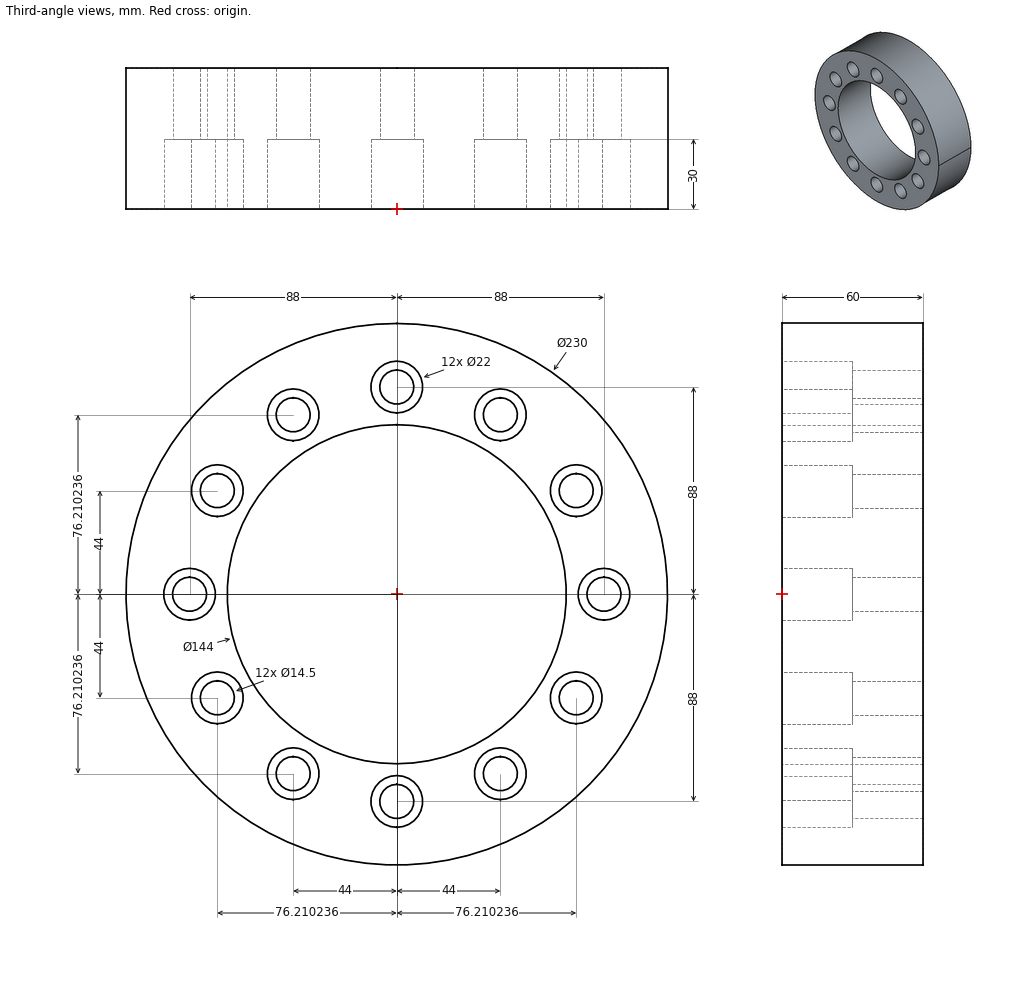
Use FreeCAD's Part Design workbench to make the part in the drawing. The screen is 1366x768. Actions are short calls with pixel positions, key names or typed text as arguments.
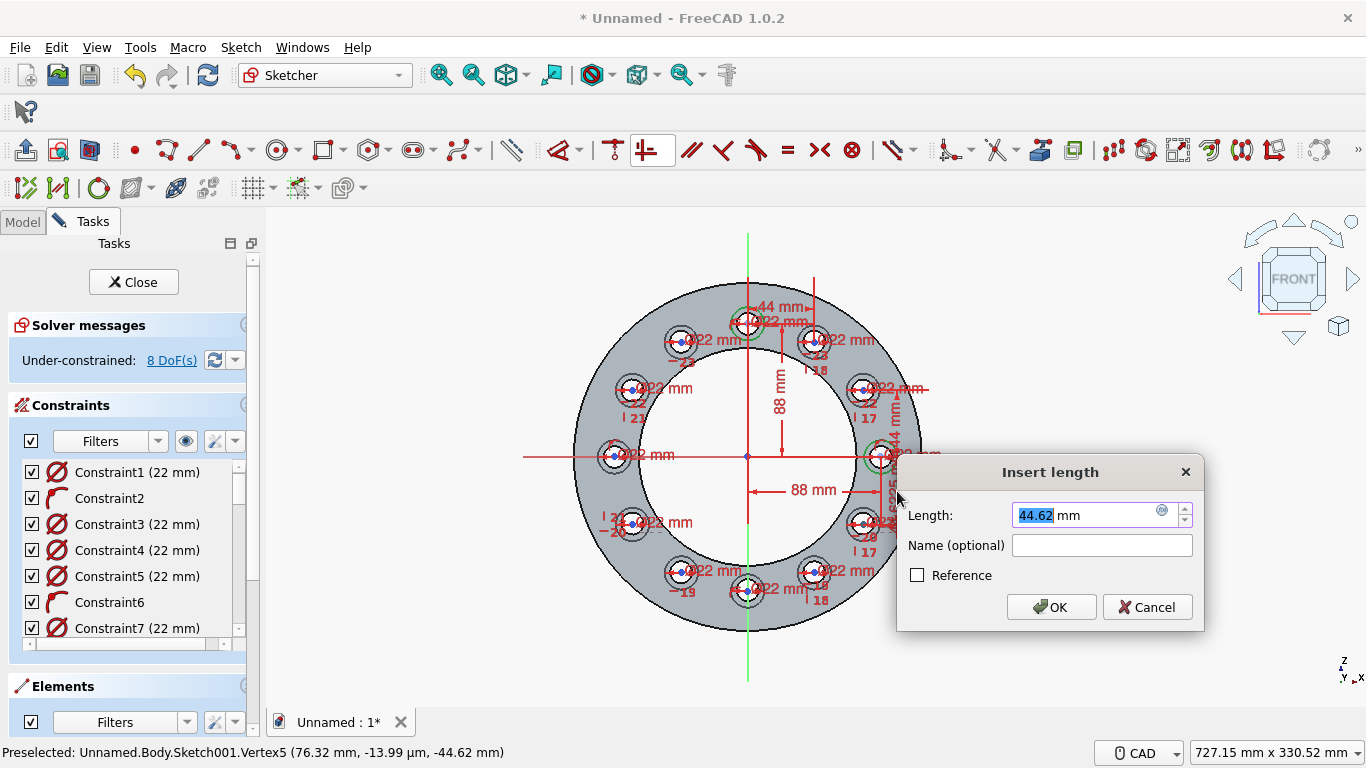
text(44)
key(Return)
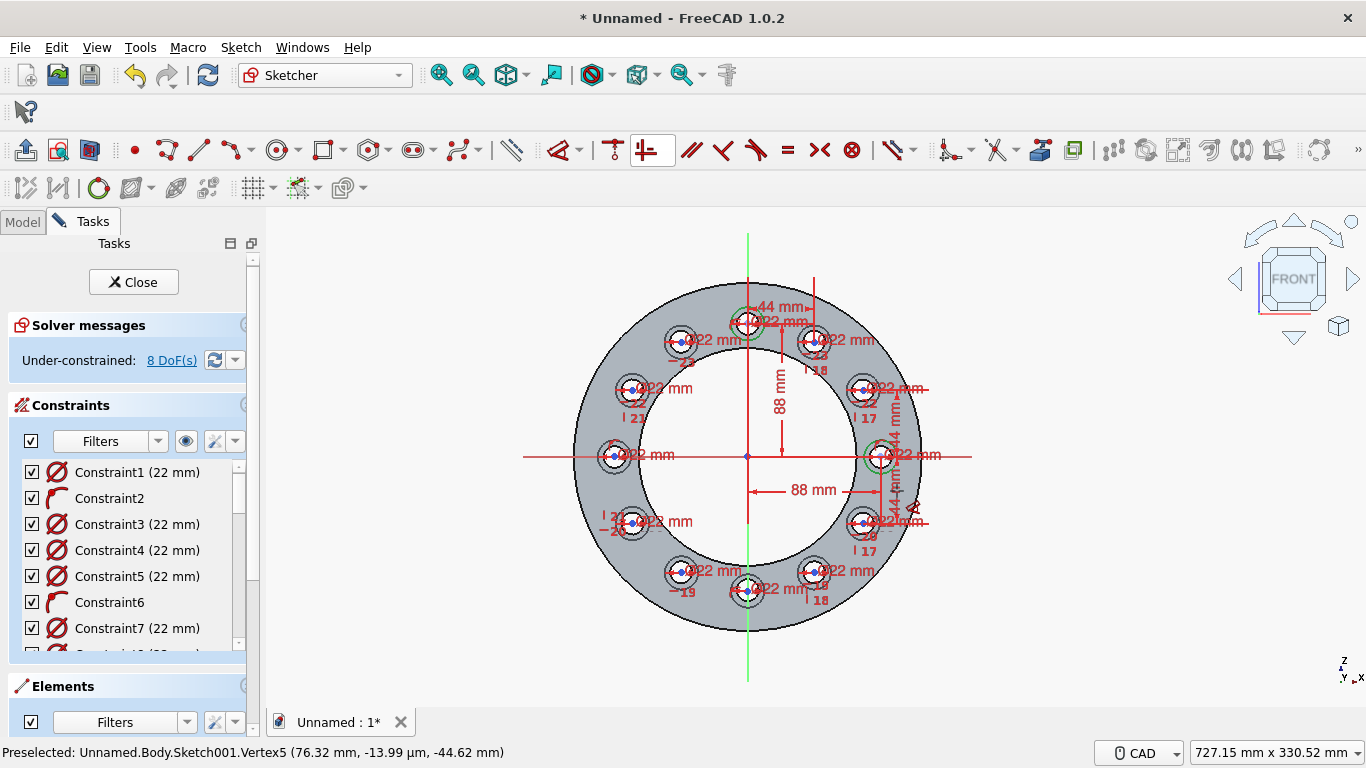
click(748, 591)
click(782, 524)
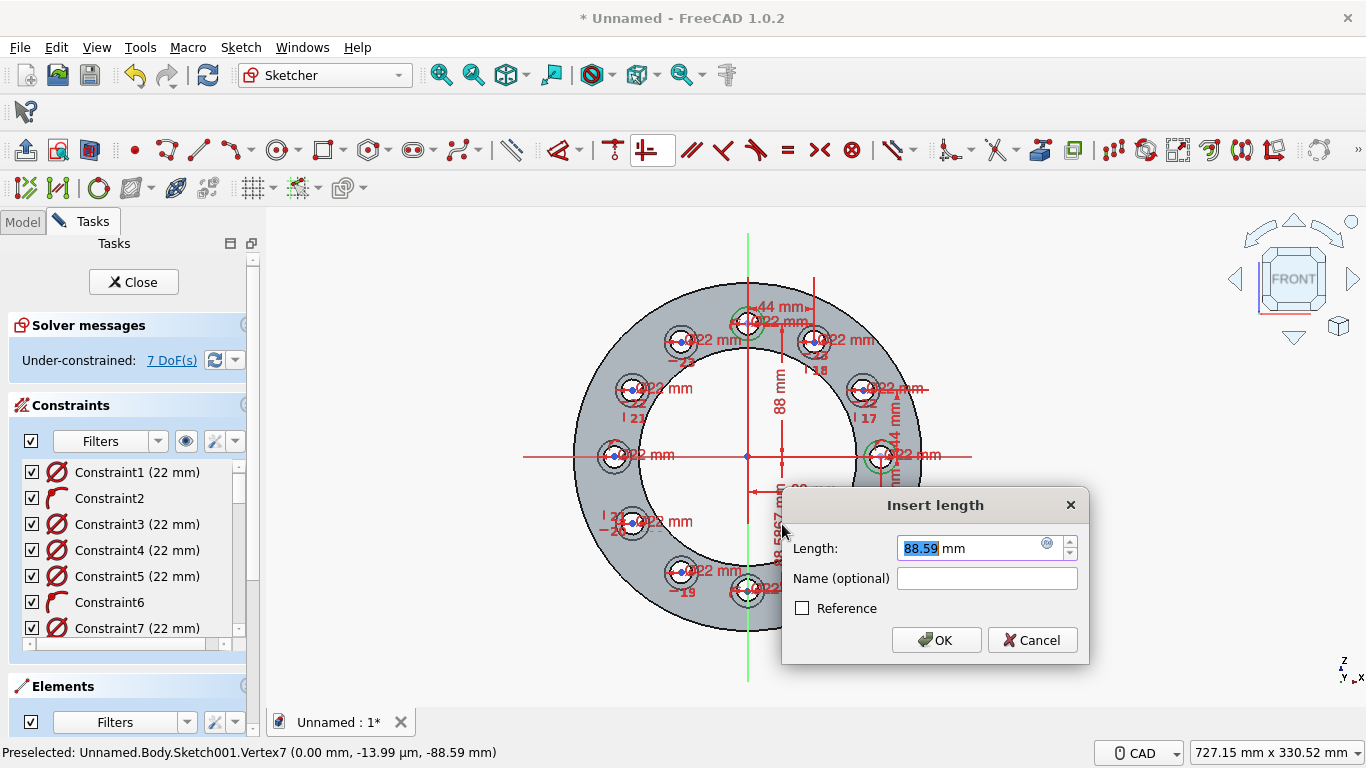
text(88)
key(Return)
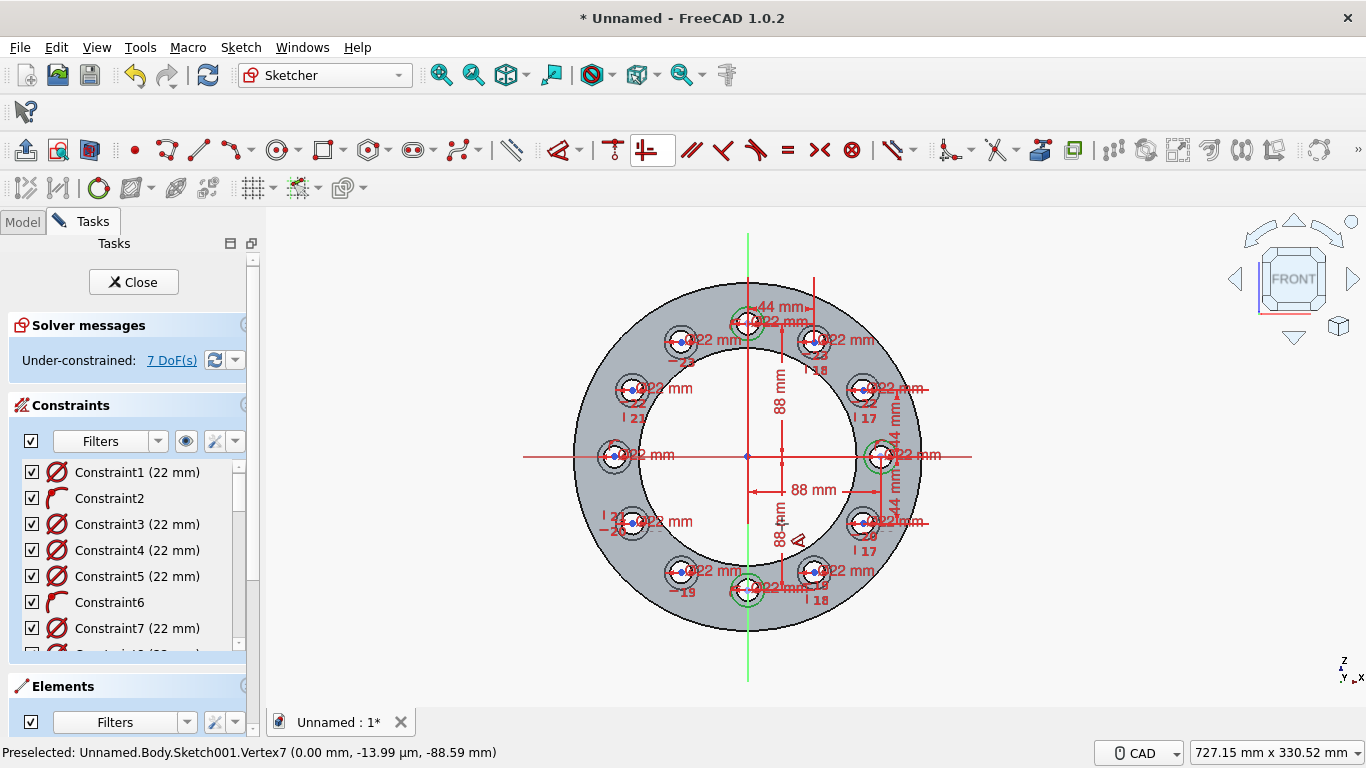
click(681, 573)
click(715, 607)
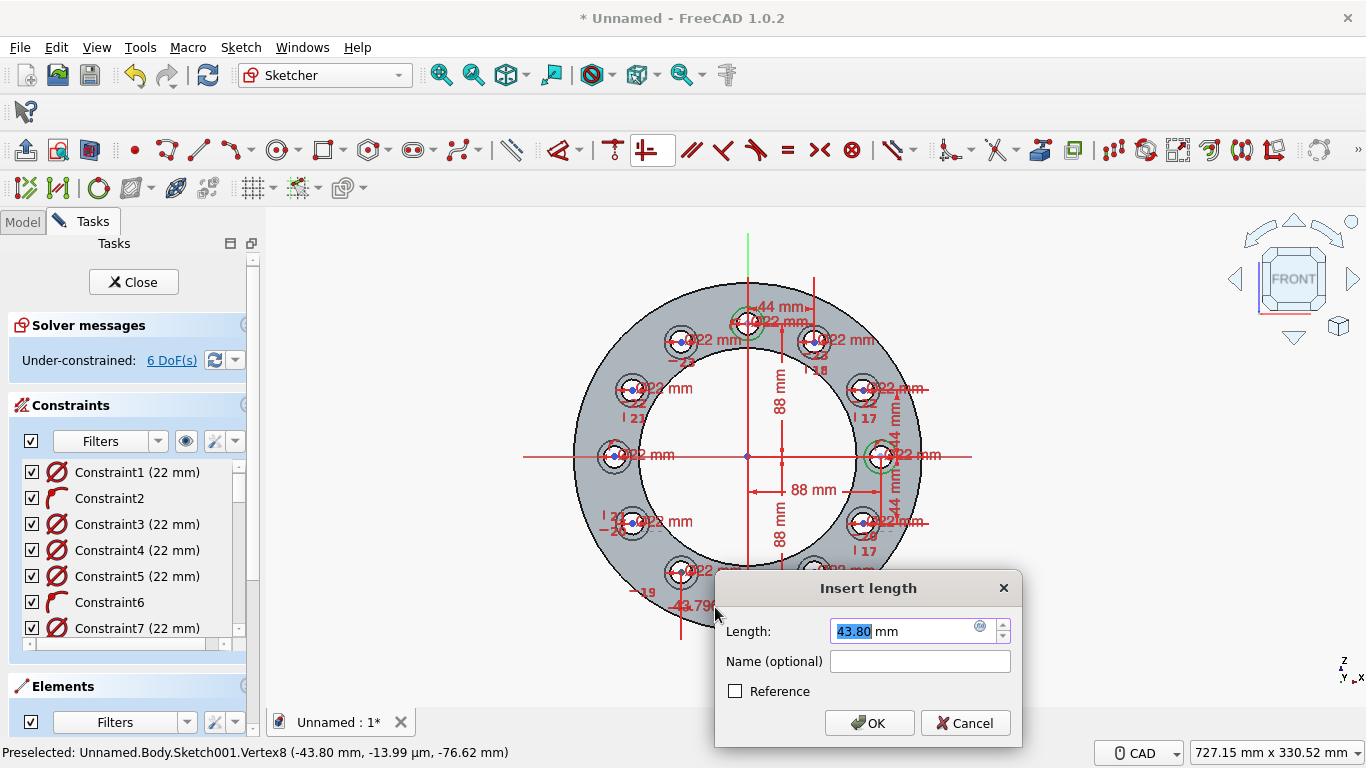
text(44)
key(Return)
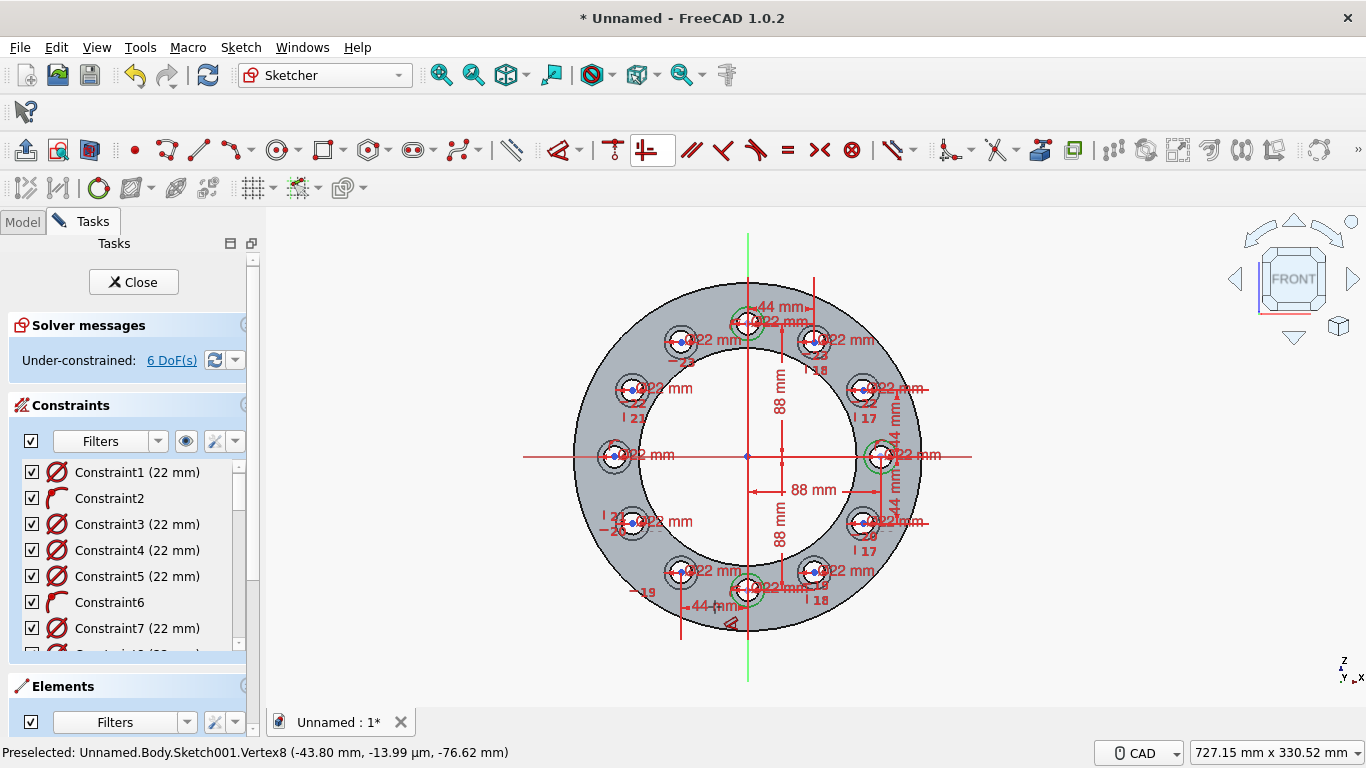
click(614, 457)
click(681, 491)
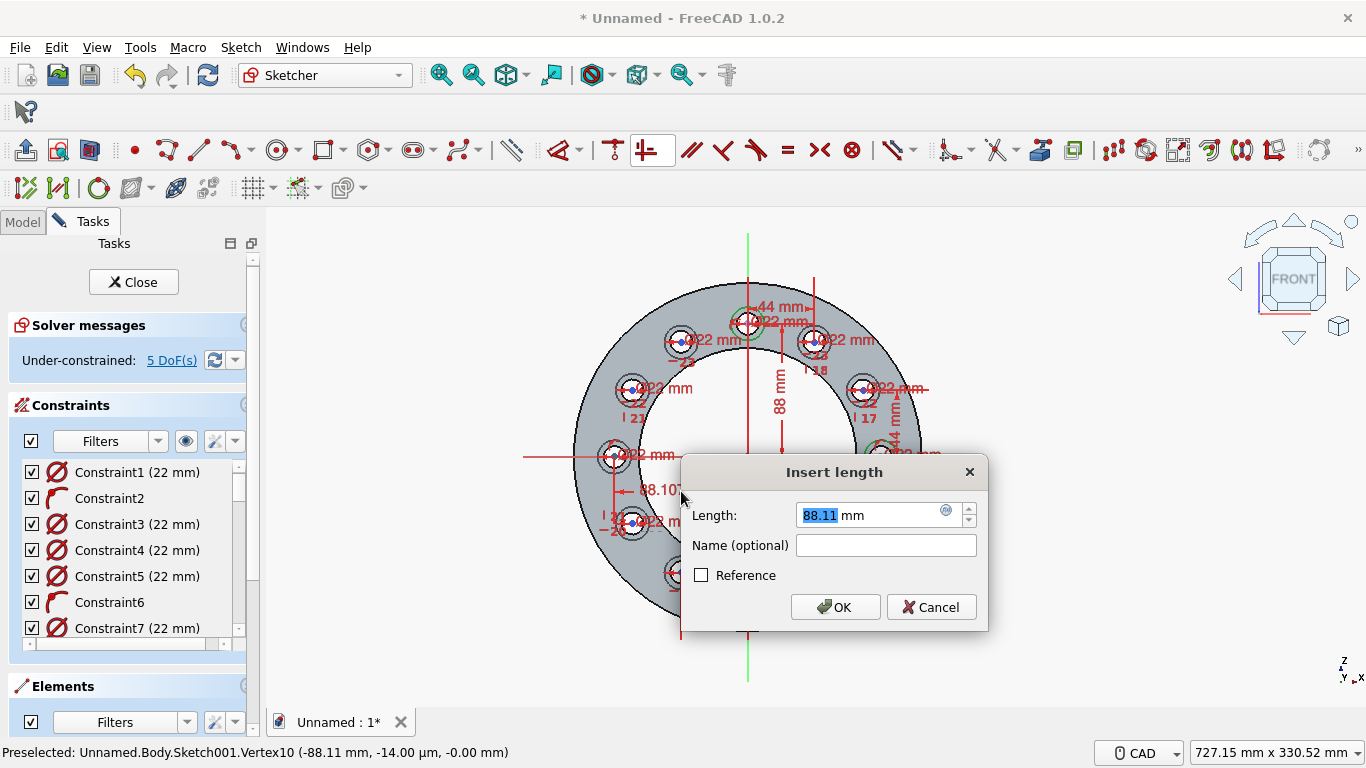
text(88)
key(Return)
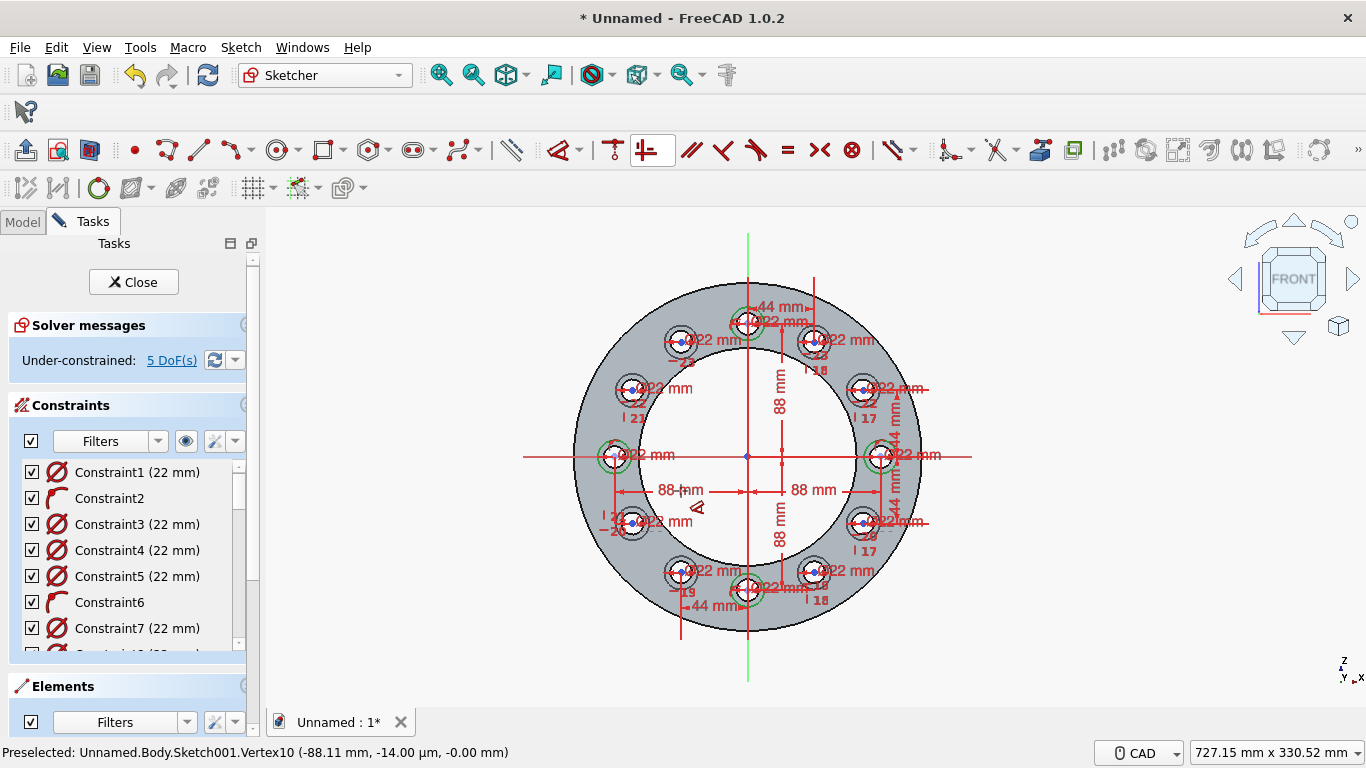
click(681, 342)
click(699, 308)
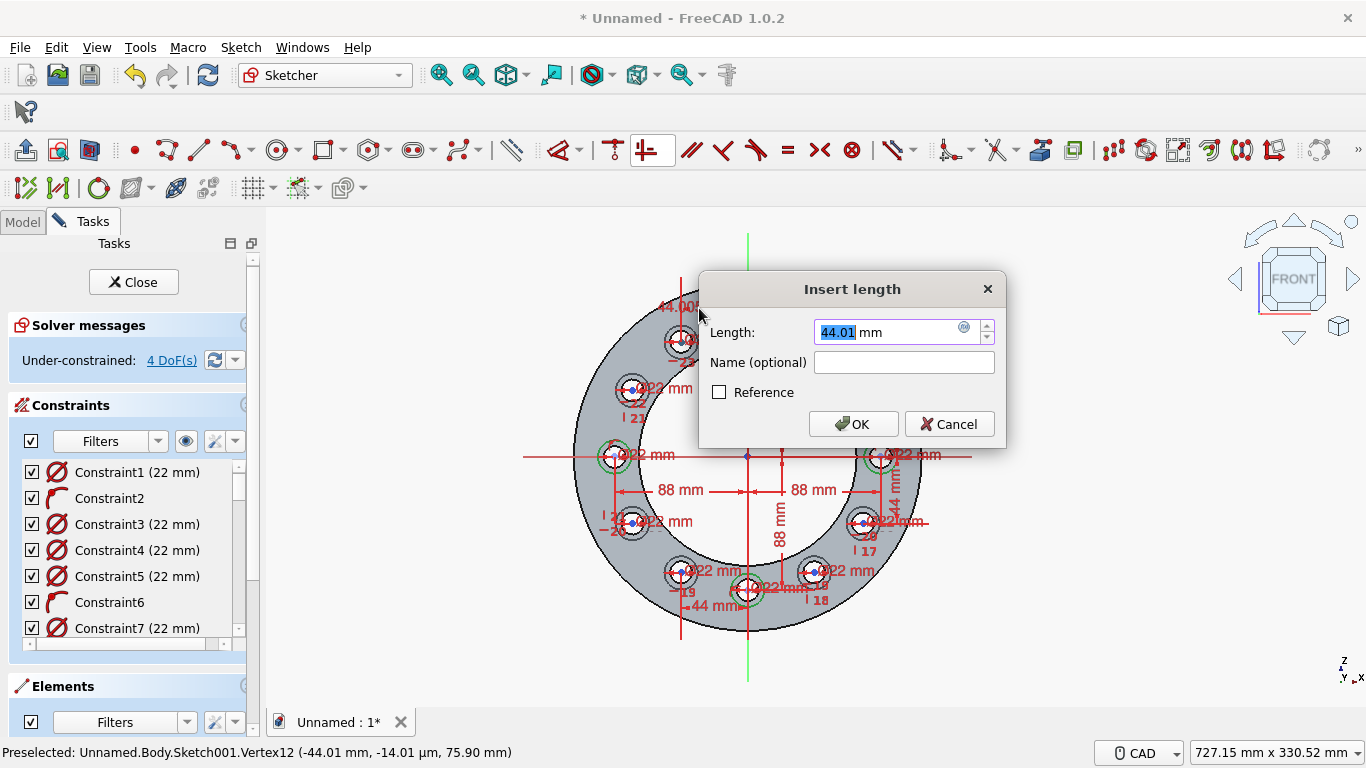
text(44)
key(Return)